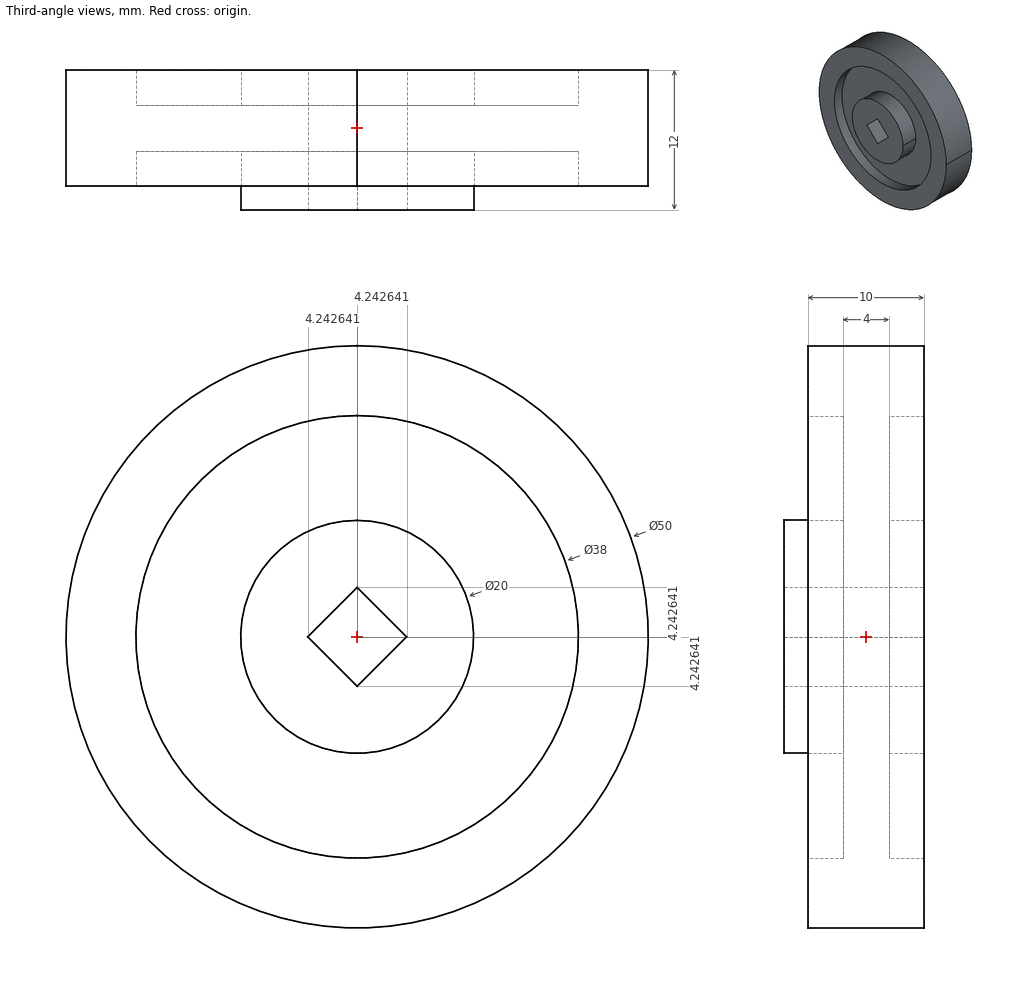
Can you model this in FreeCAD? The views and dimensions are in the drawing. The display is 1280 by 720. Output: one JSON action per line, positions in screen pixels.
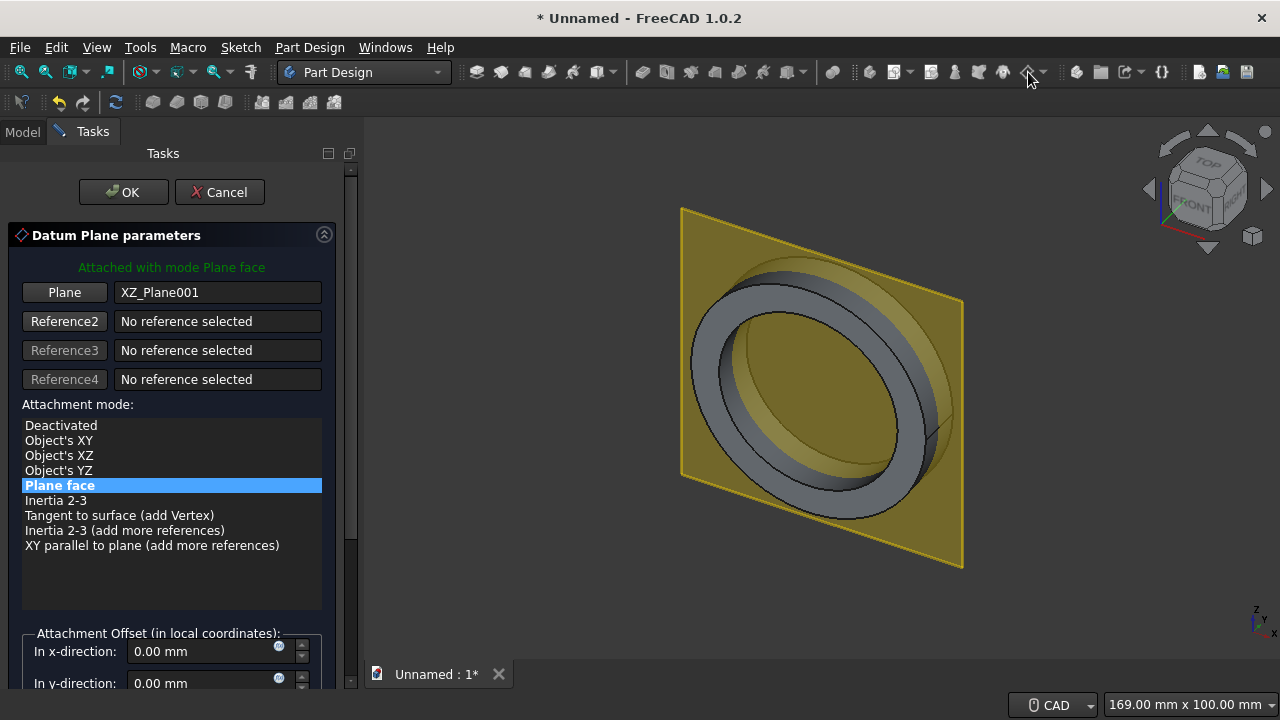
{"action": "scroll", "coordinate": [351, 426], "scroll_direction": "down", "scroll_amount": 2}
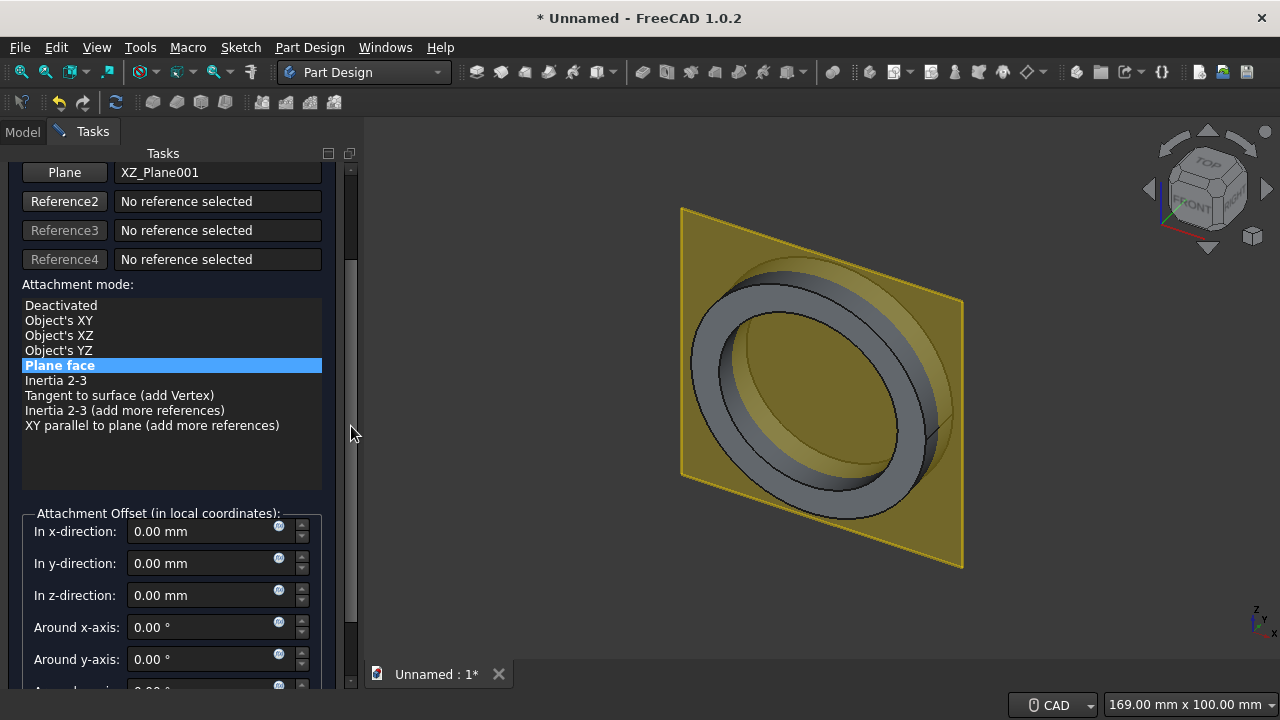
{"action": "triple_click", "coordinate": [210, 595]}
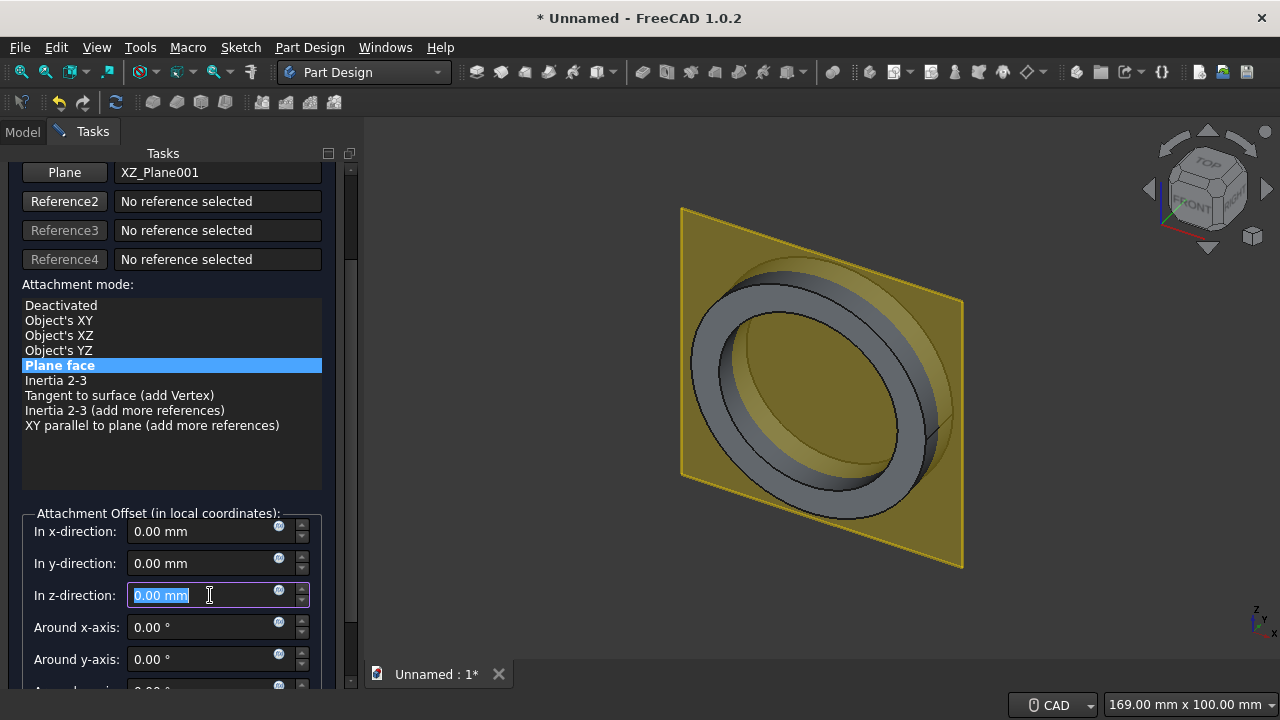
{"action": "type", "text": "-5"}
{"action": "key", "text": "Tab"}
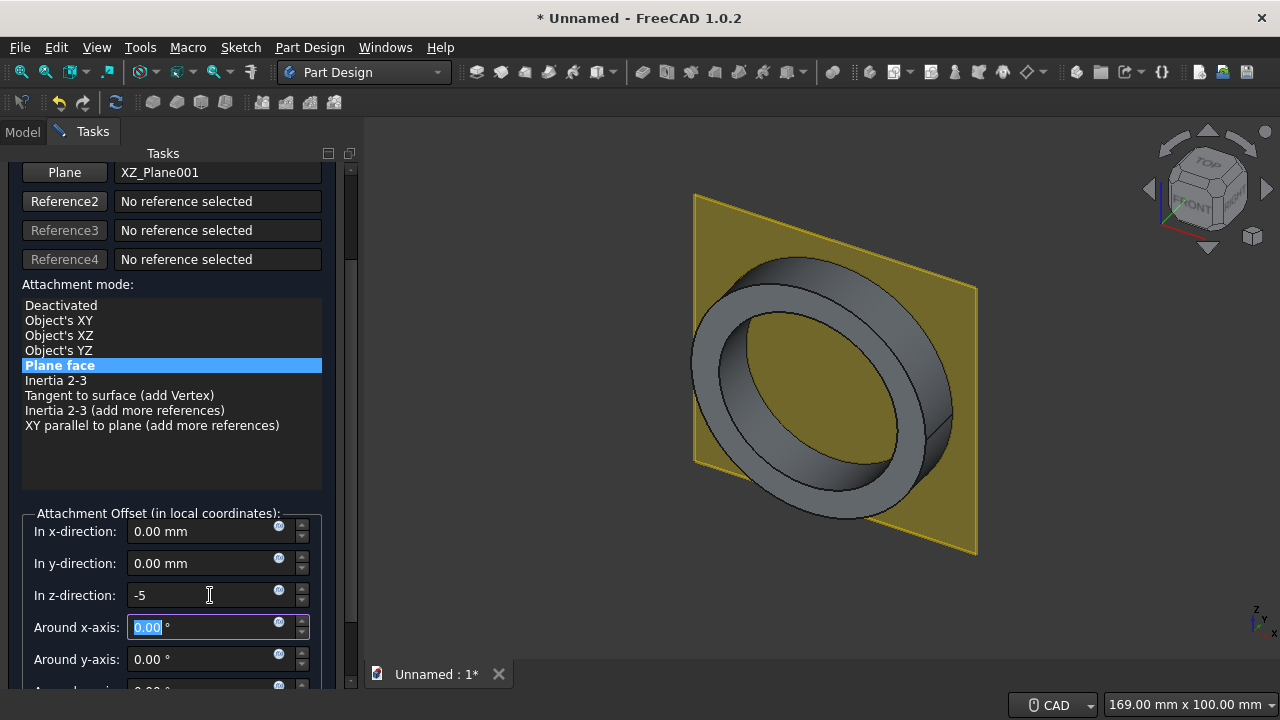
{"action": "scroll", "coordinate": [351, 426], "scroll_direction": "up", "scroll_amount": 3}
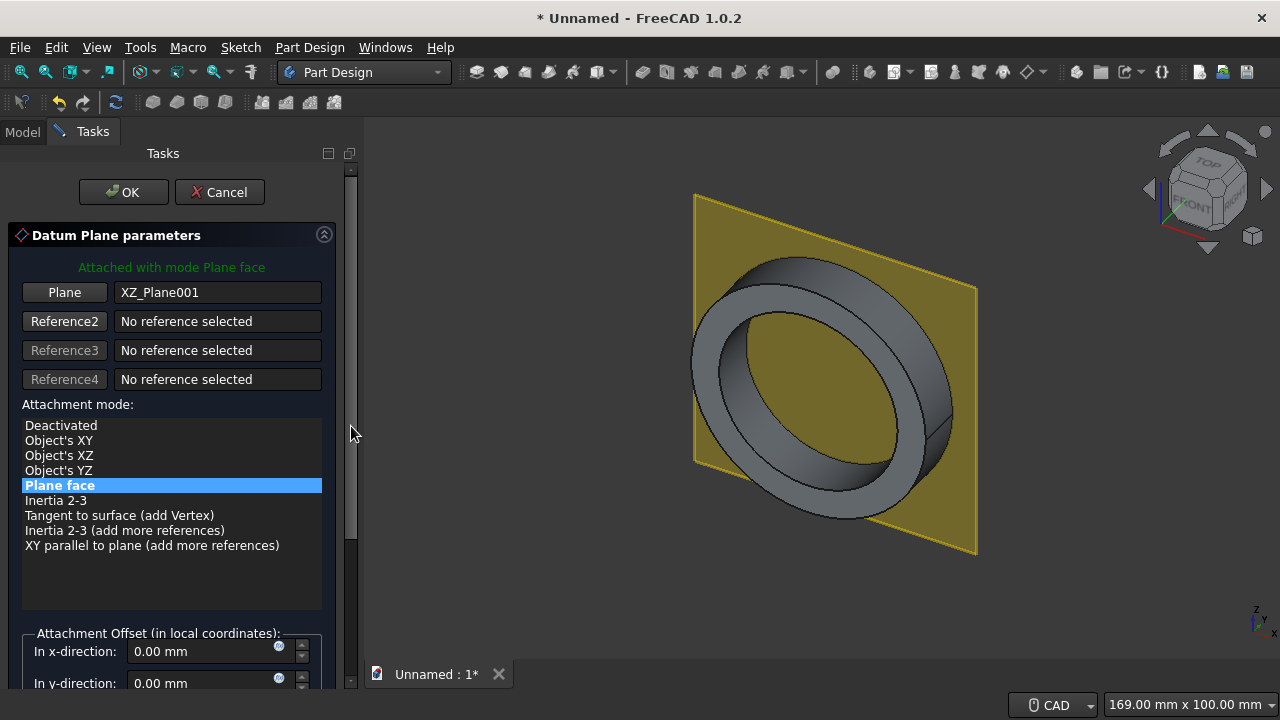
{"action": "left_click", "coordinate": [124, 192]}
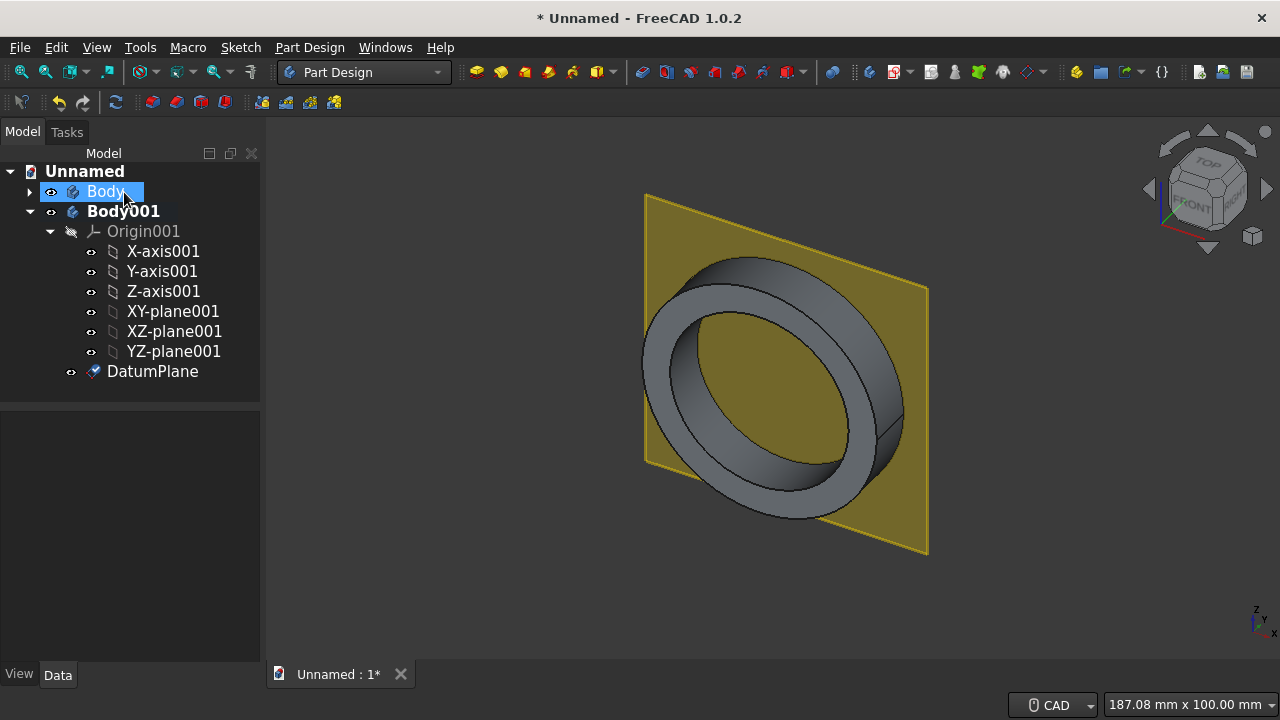
{"action": "left_click", "coordinate": [116, 372]}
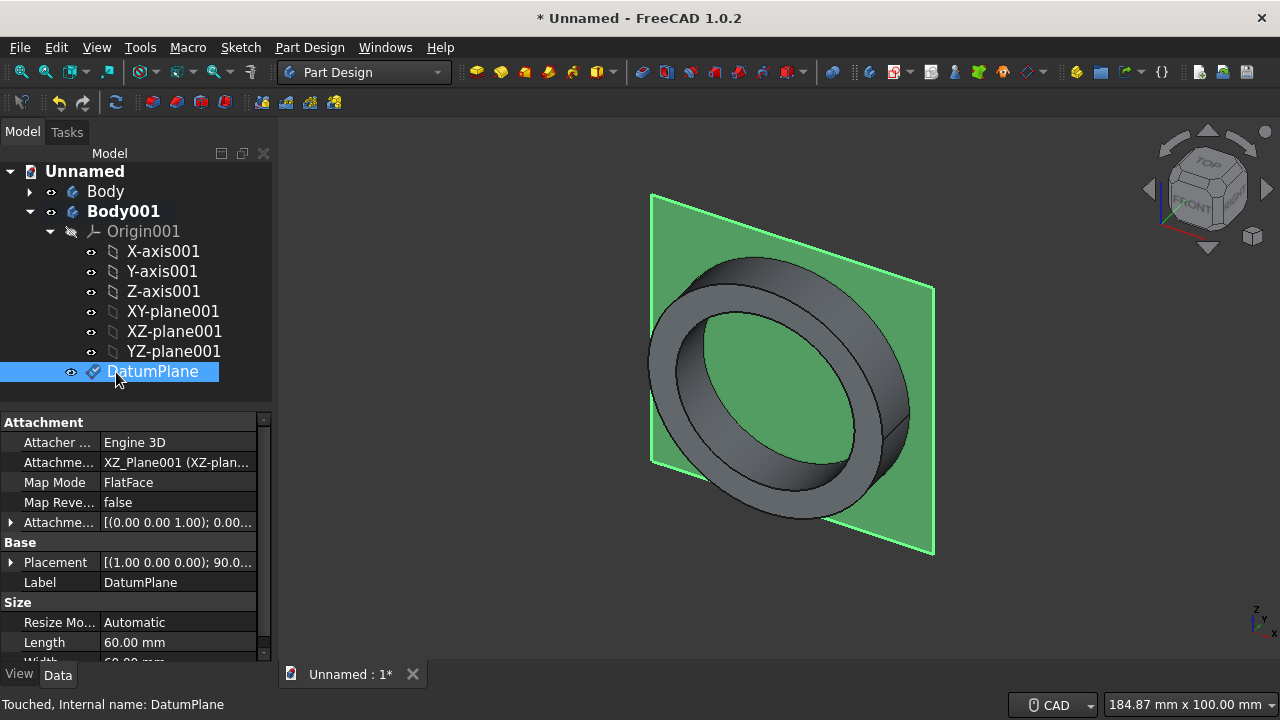
{"action": "left_click", "coordinate": [894, 72]}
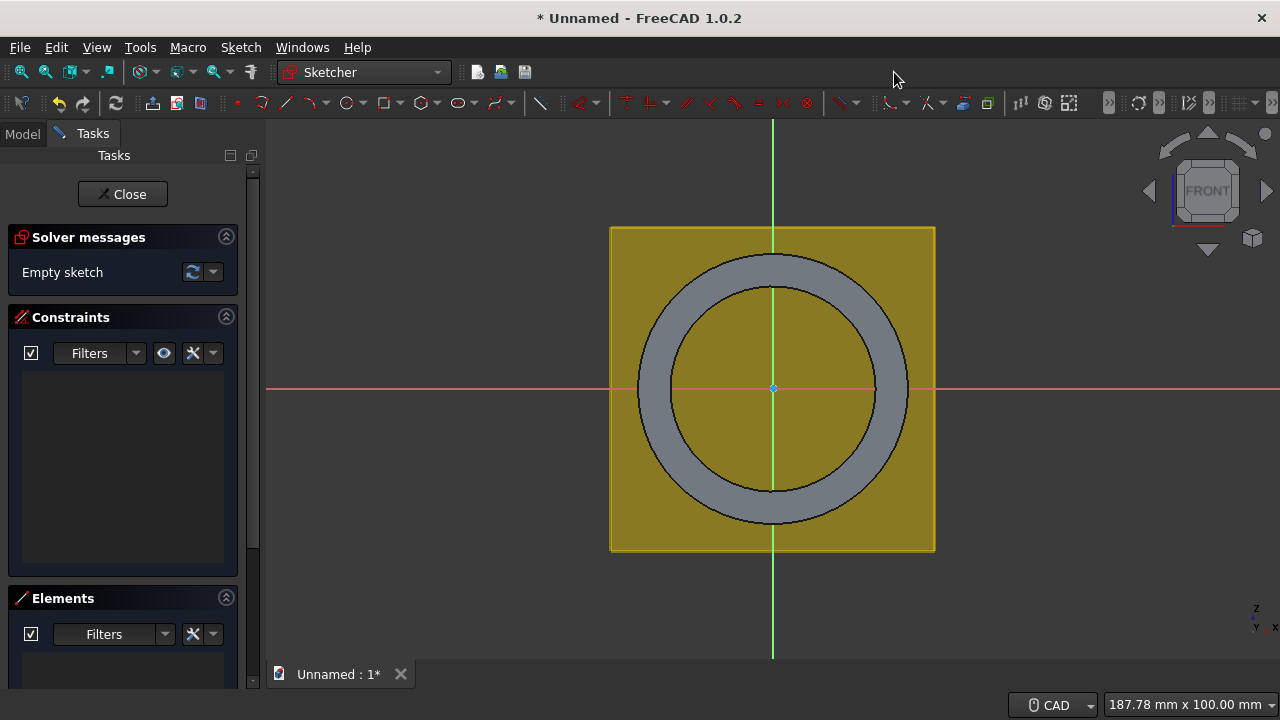
{"action": "scroll", "coordinate": [803, 389], "scroll_direction": "up", "scroll_amount": 6}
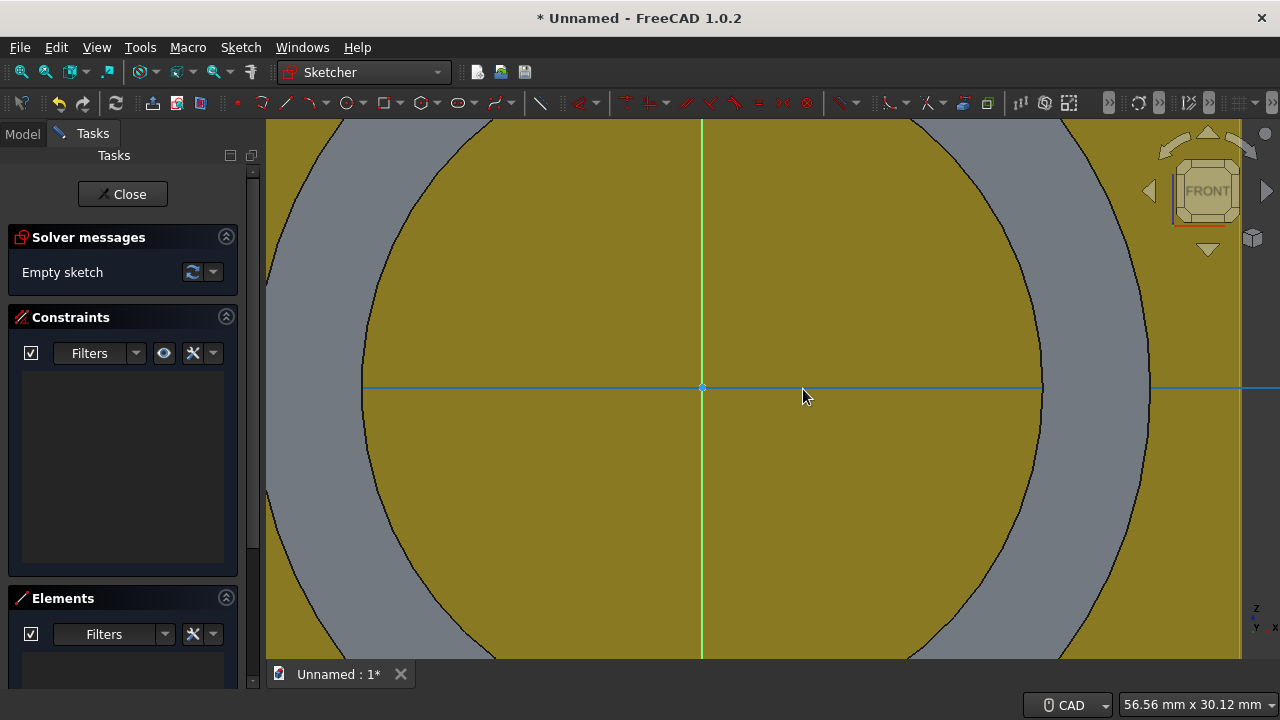
{"action": "left_click", "coordinate": [348, 104]}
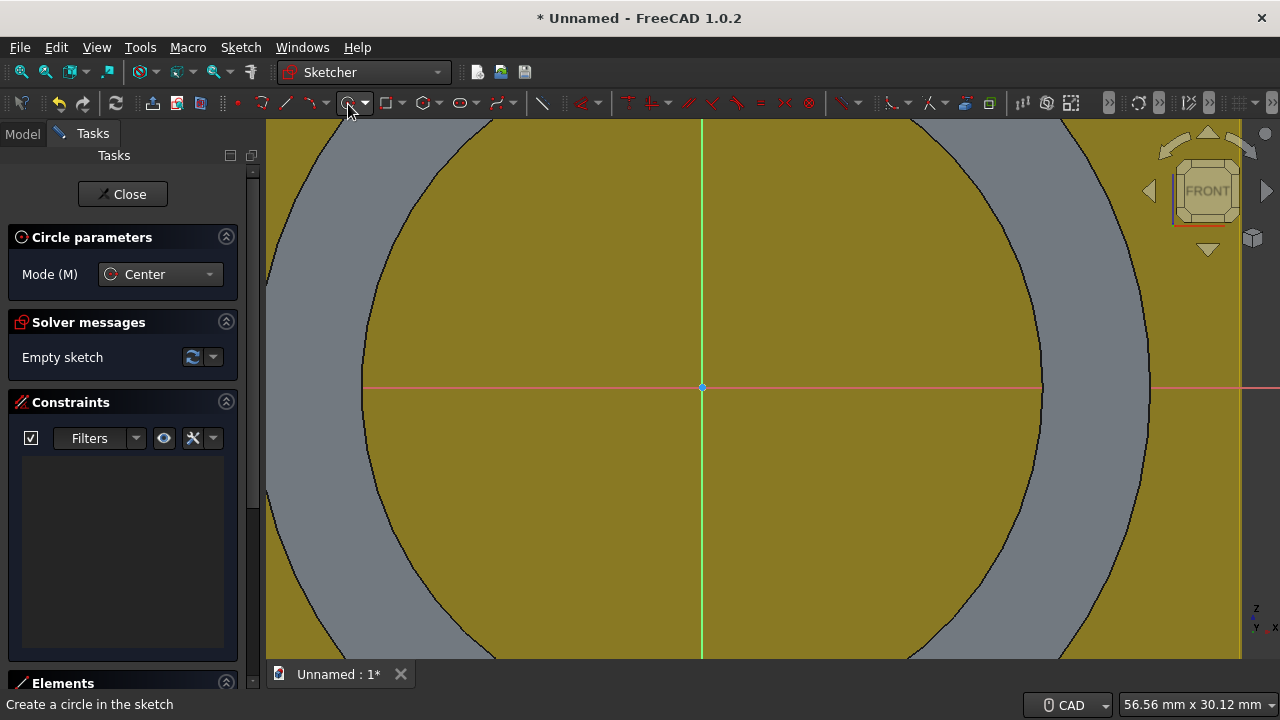
{"action": "left_click", "coordinate": [702, 388]}
{"action": "left_click", "coordinate": [829, 261]}
{"action": "key", "text": "Escape"}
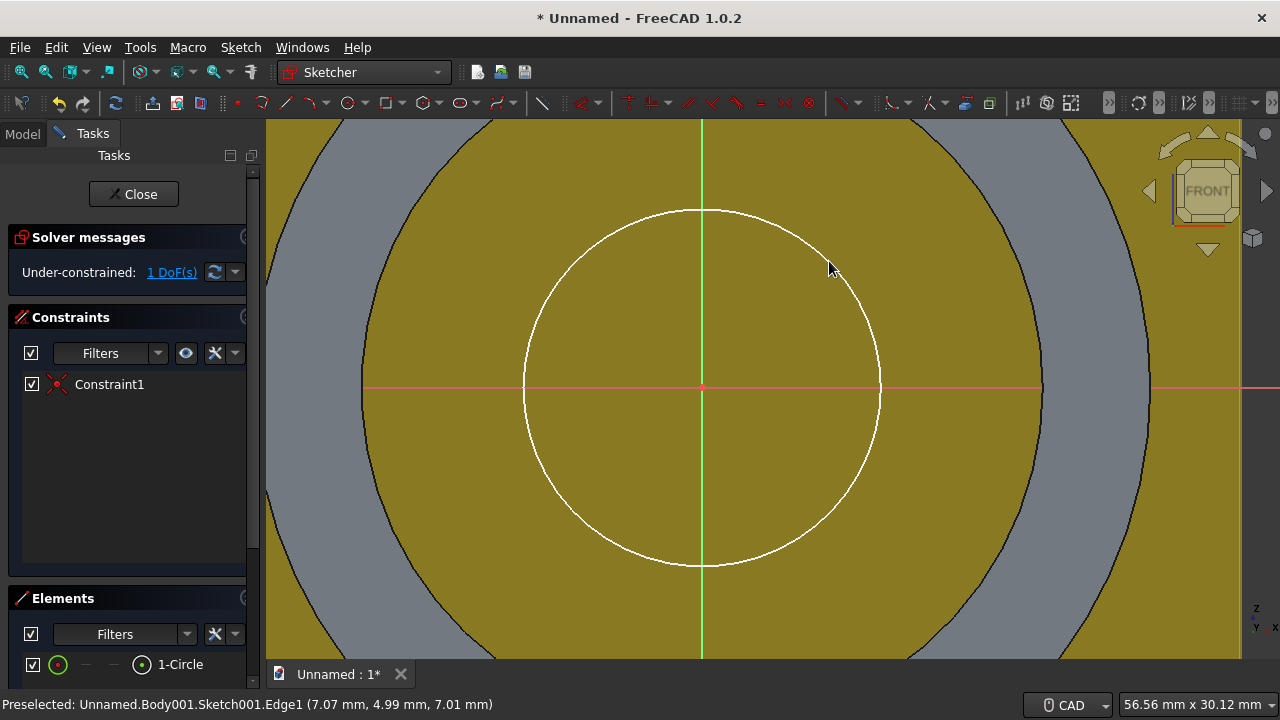
{"action": "left_click", "coordinate": [582, 104]}